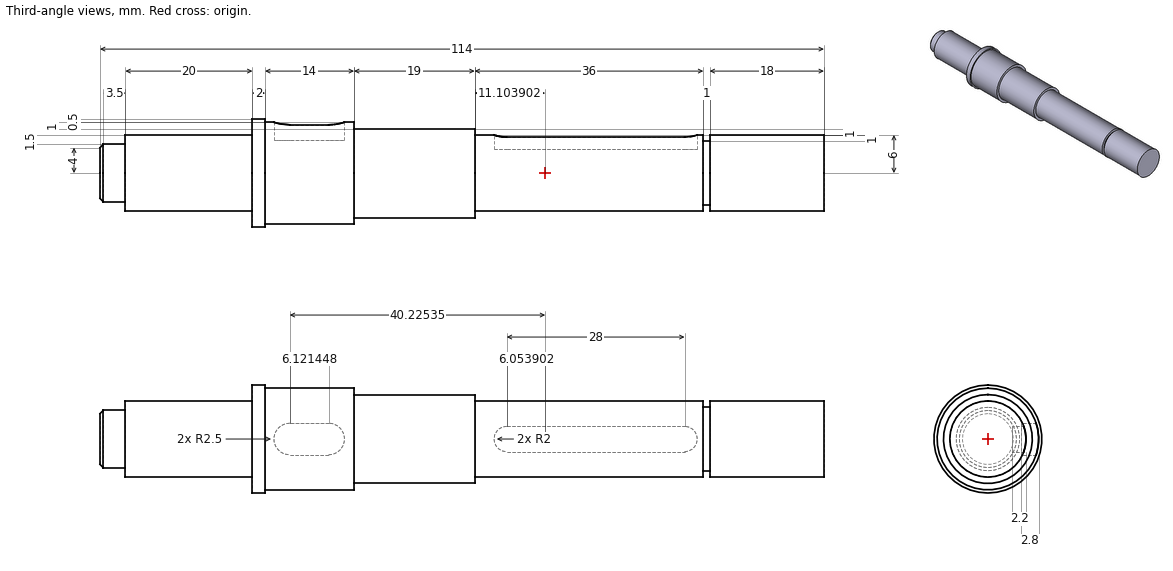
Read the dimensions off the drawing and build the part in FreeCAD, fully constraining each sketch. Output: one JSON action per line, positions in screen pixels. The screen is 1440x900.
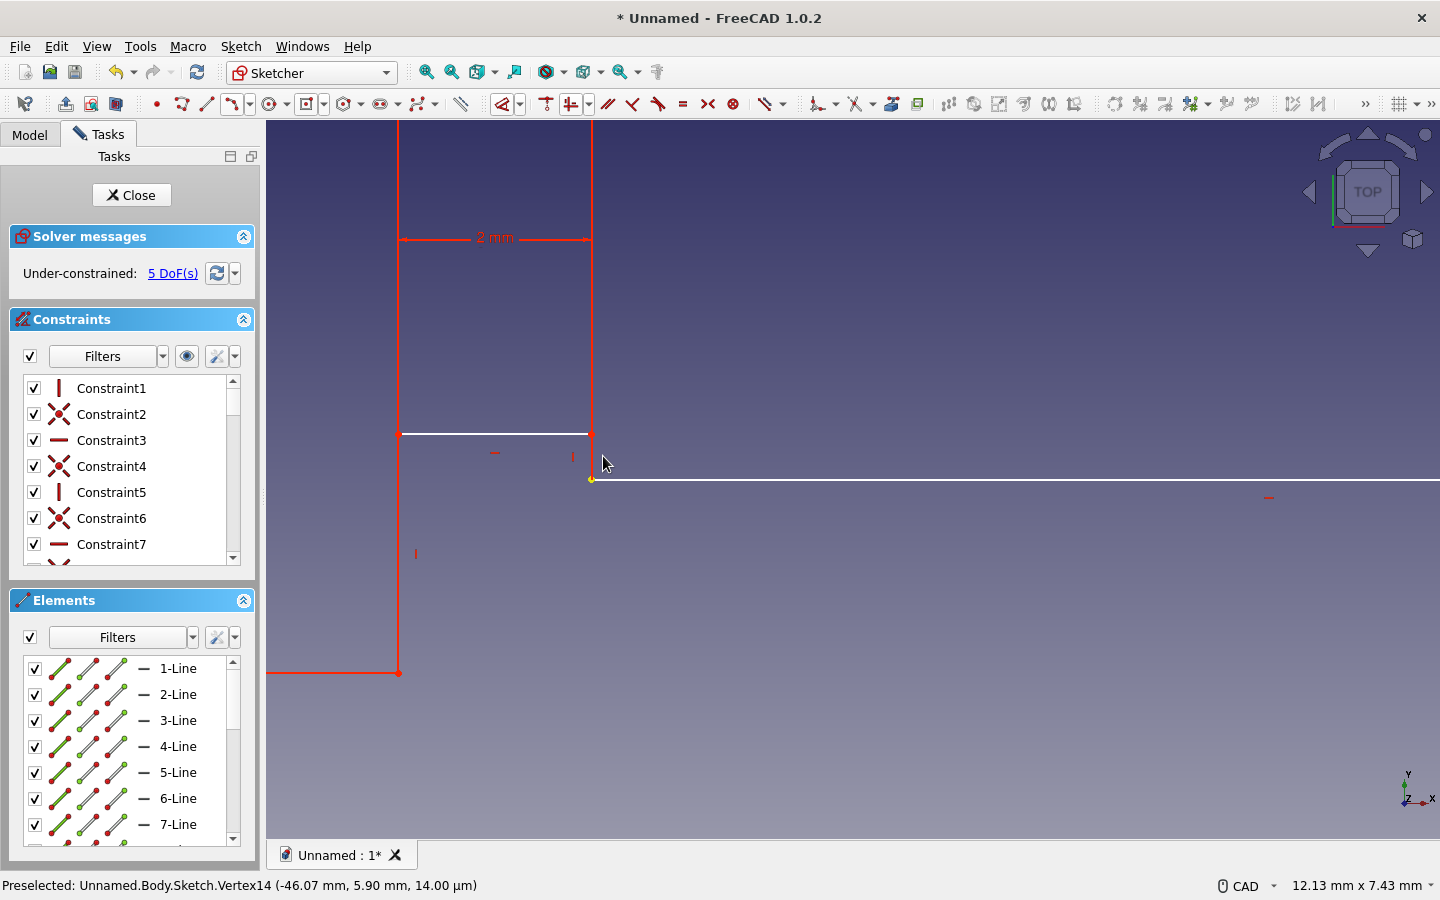
{"action": "left_click", "coordinate": [592, 457]}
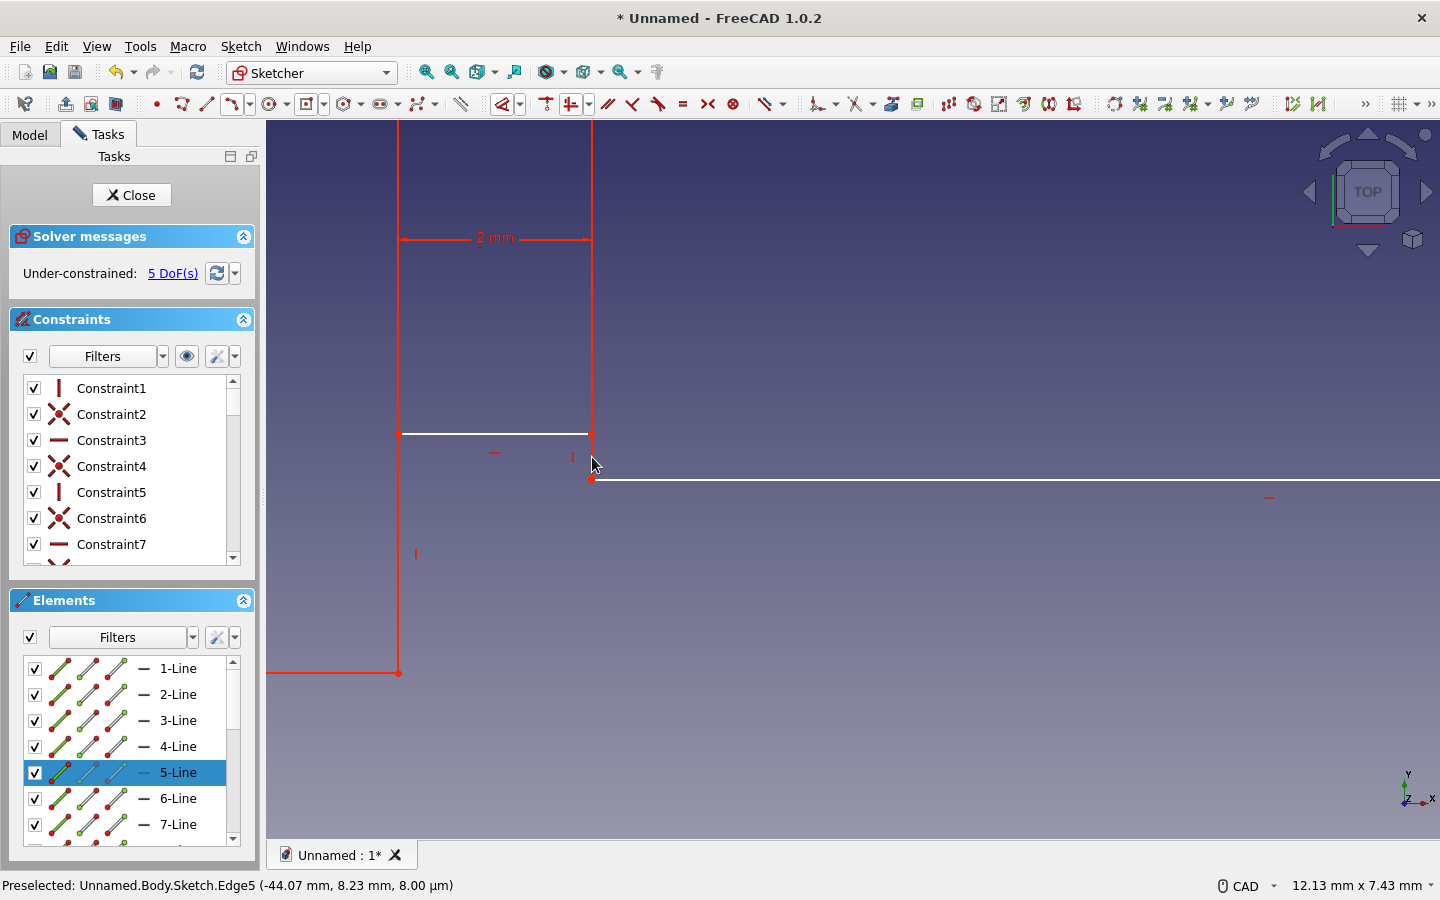
{"action": "left_click", "coordinate": [520, 104]}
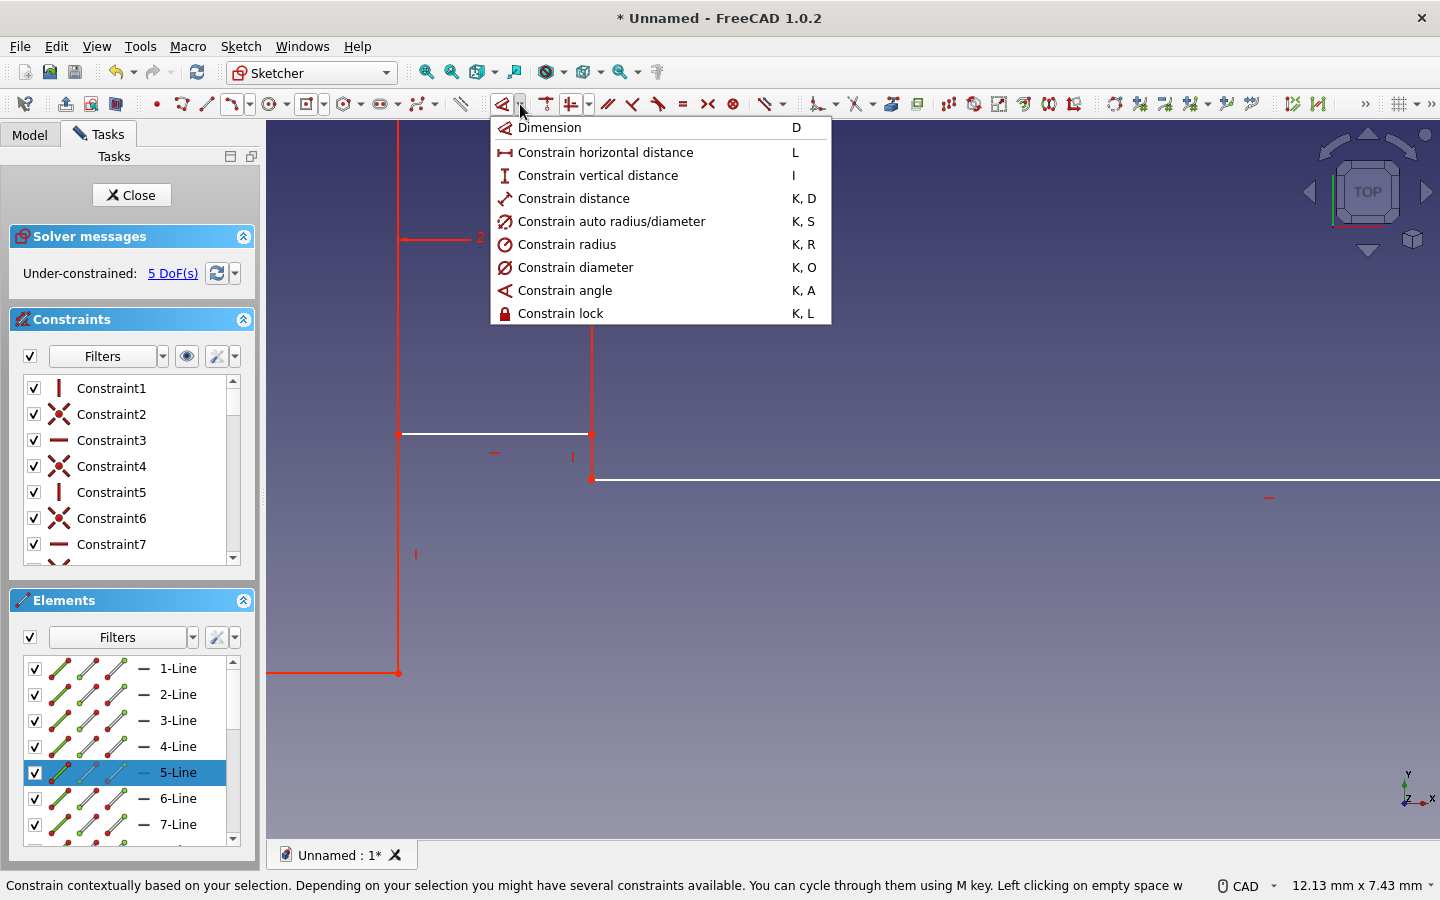
{"action": "left_click", "coordinate": [661, 176]}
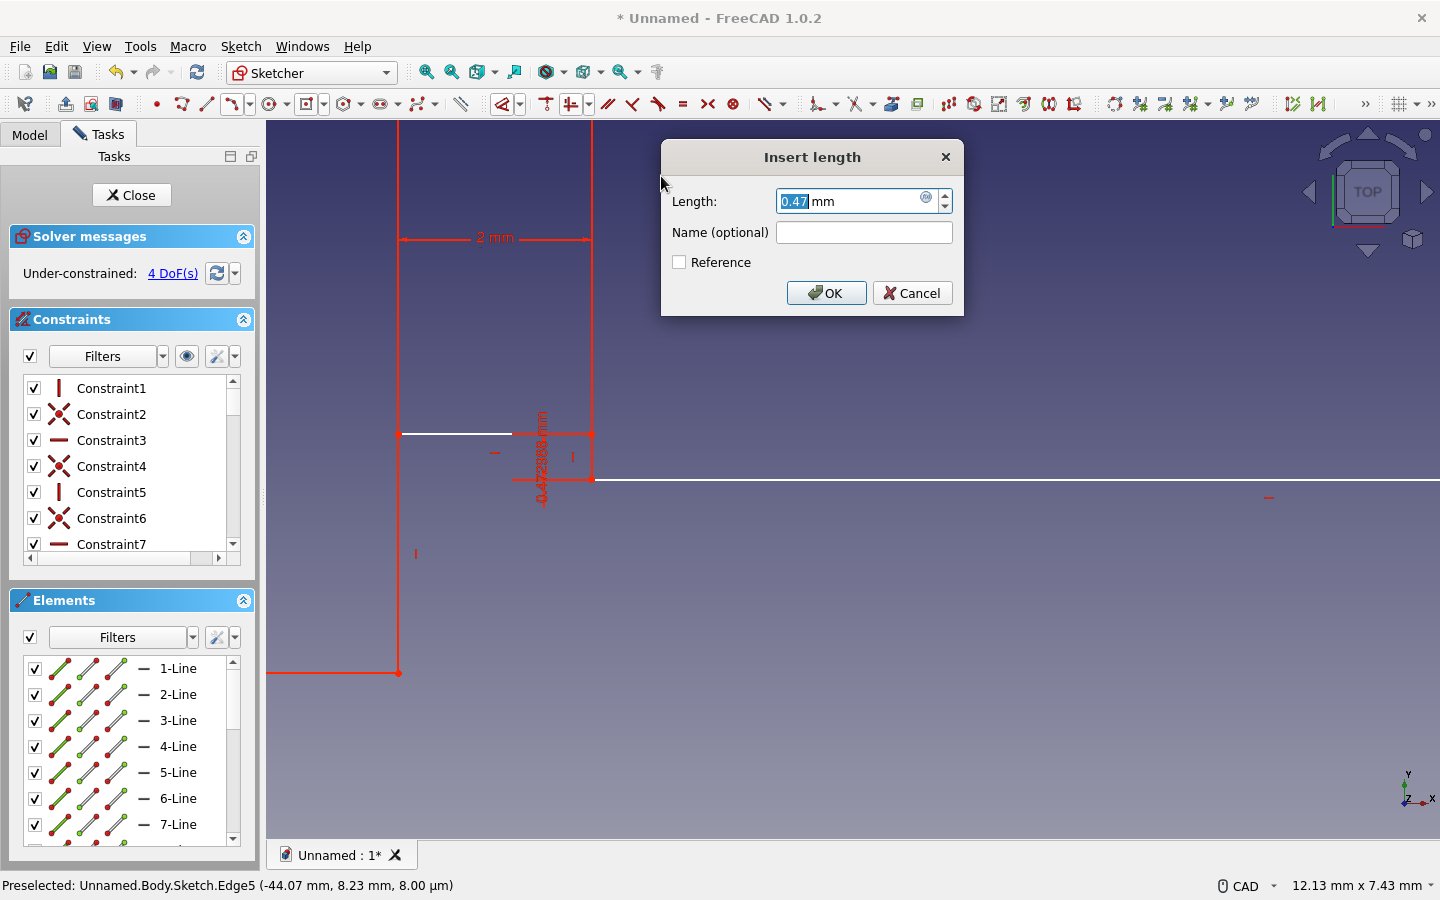
{"action": "type", "text": "0.5"}
{"action": "key", "text": "Return"}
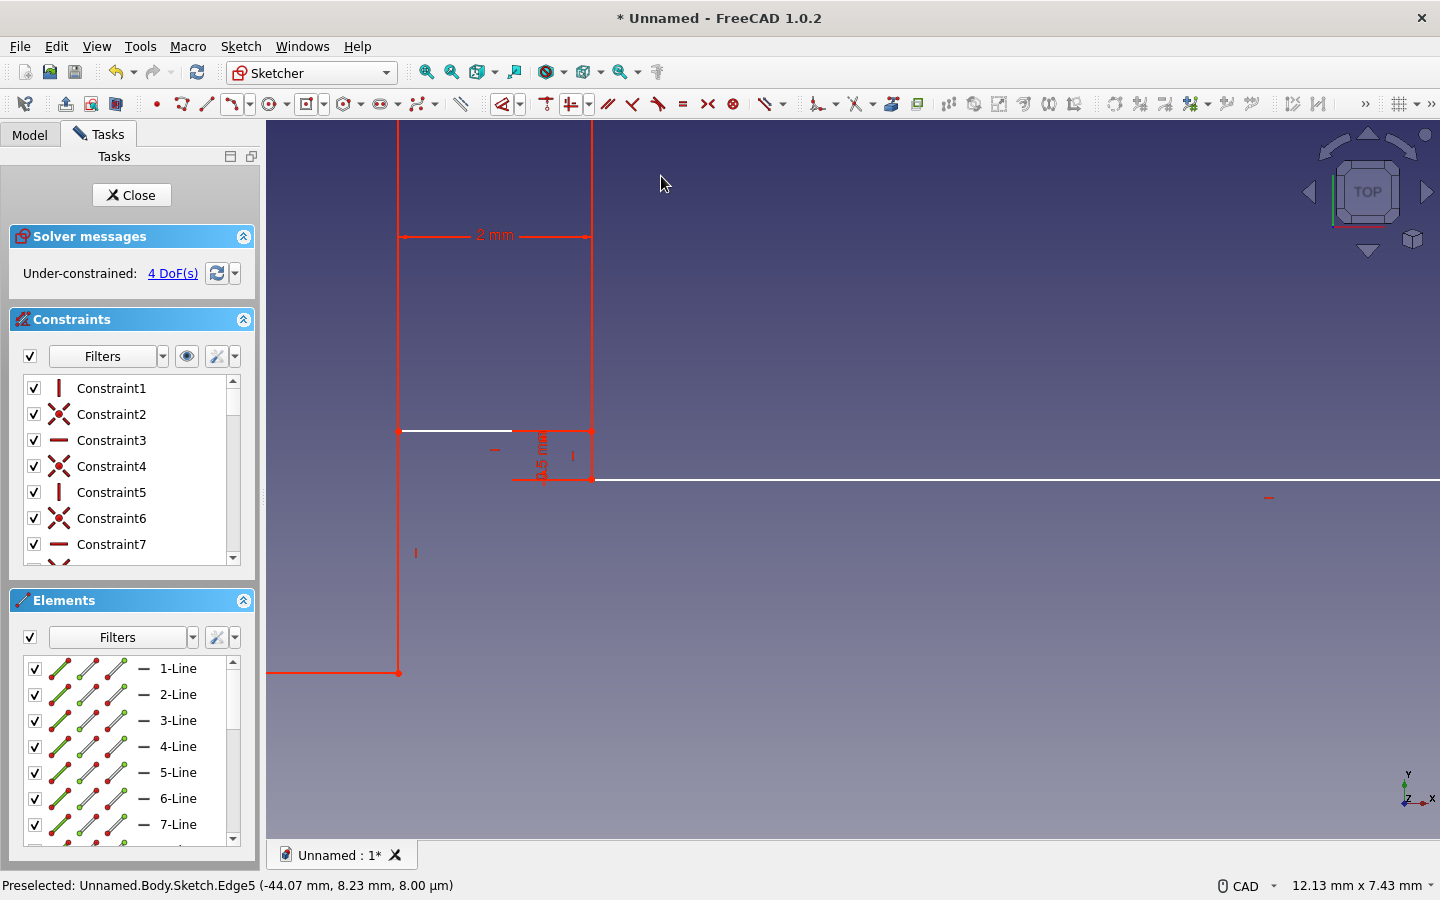
{"action": "scroll", "coordinate": [603, 456], "scroll_direction": "down", "scroll_amount": 14}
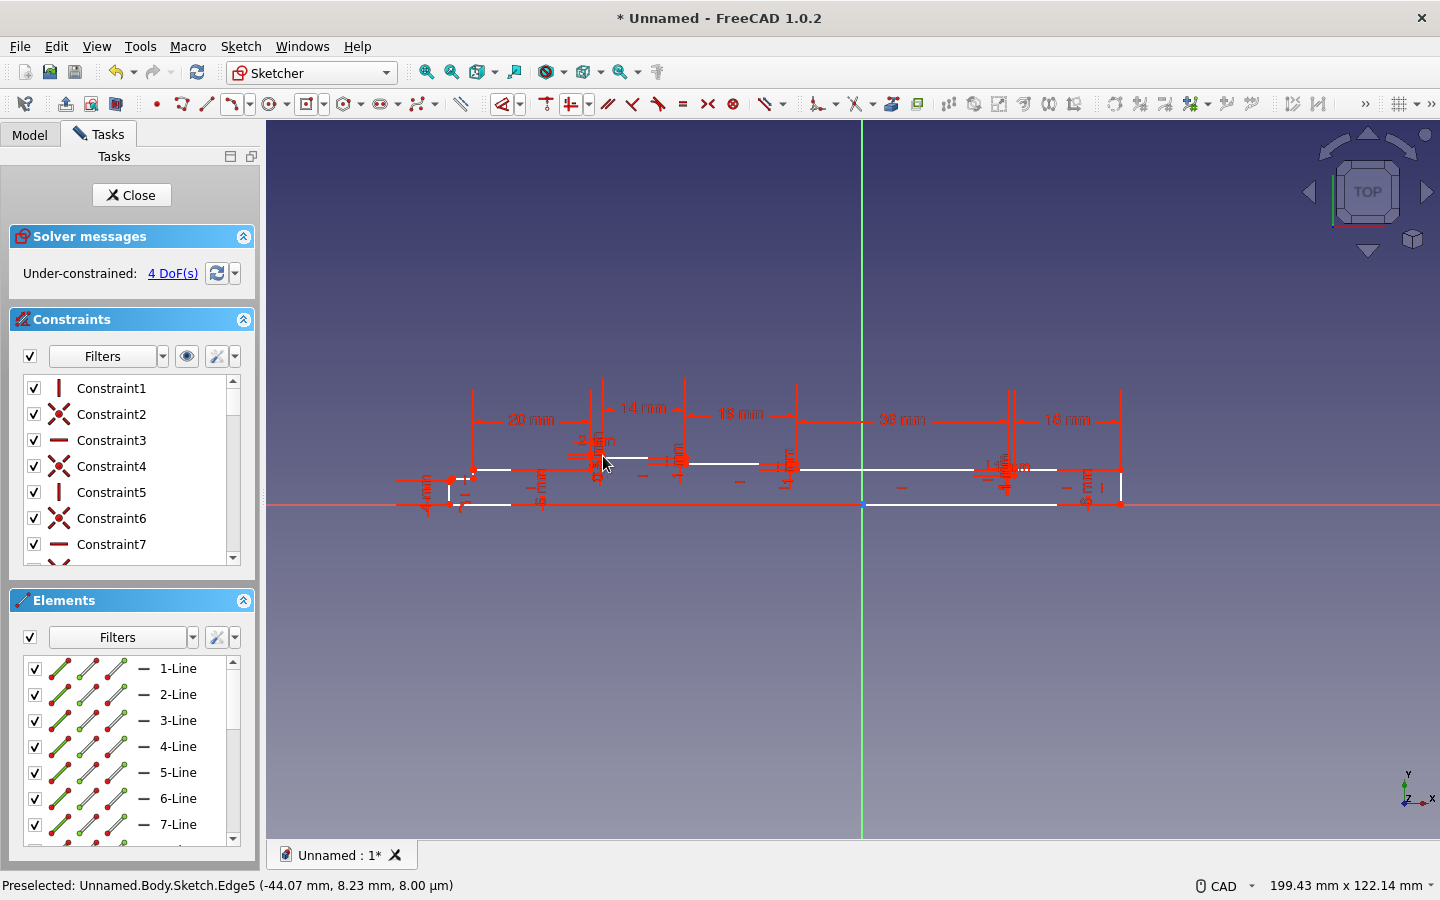
{"action": "scroll", "coordinate": [473, 472], "scroll_direction": "up", "scroll_amount": 8}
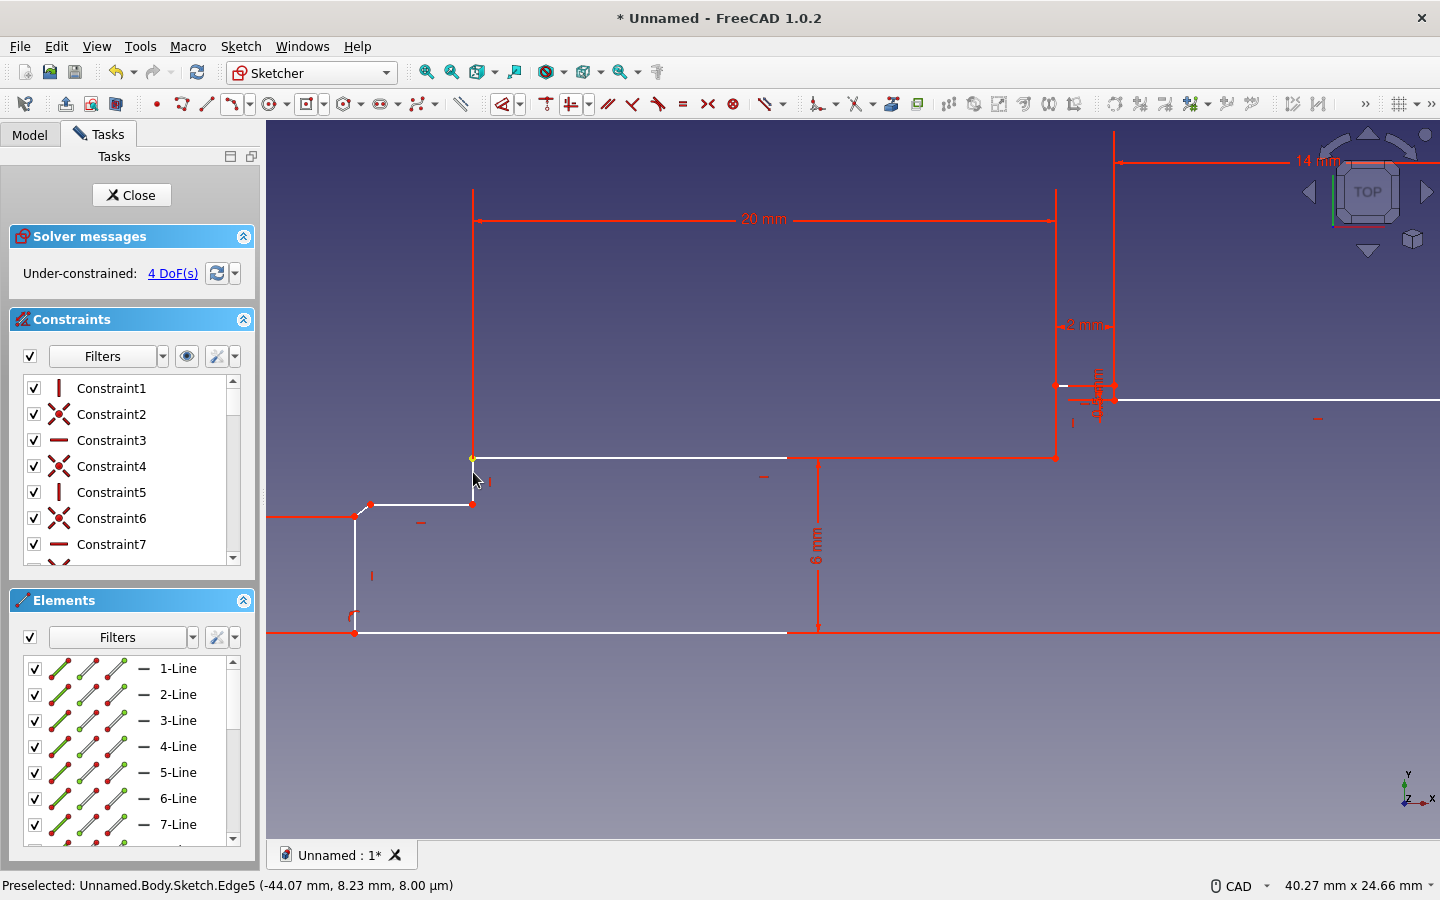
{"action": "left_click", "coordinate": [473, 472]}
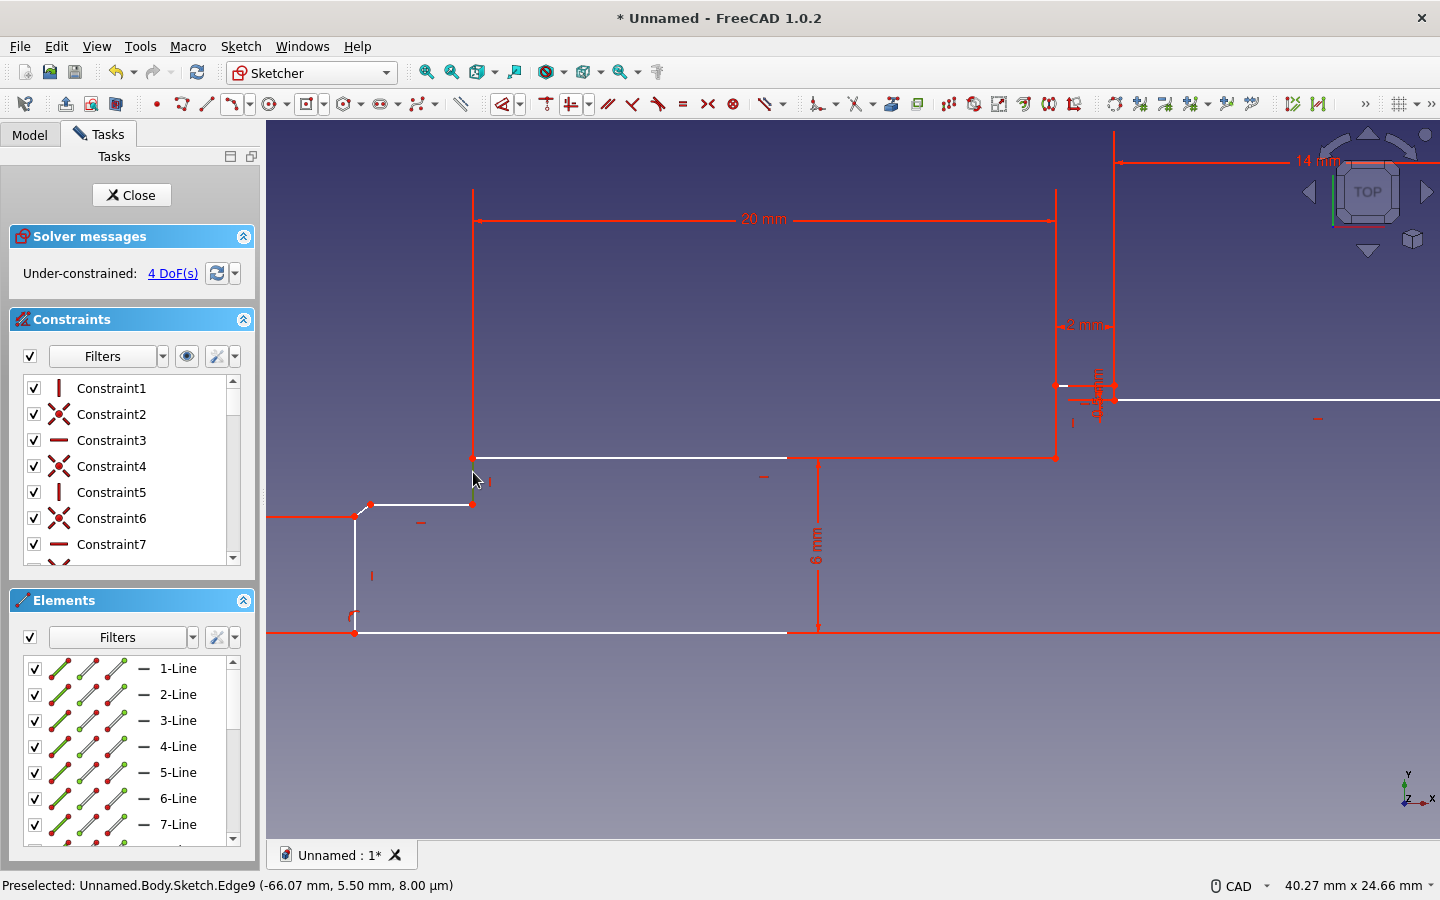
{"action": "key", "text": "i"}